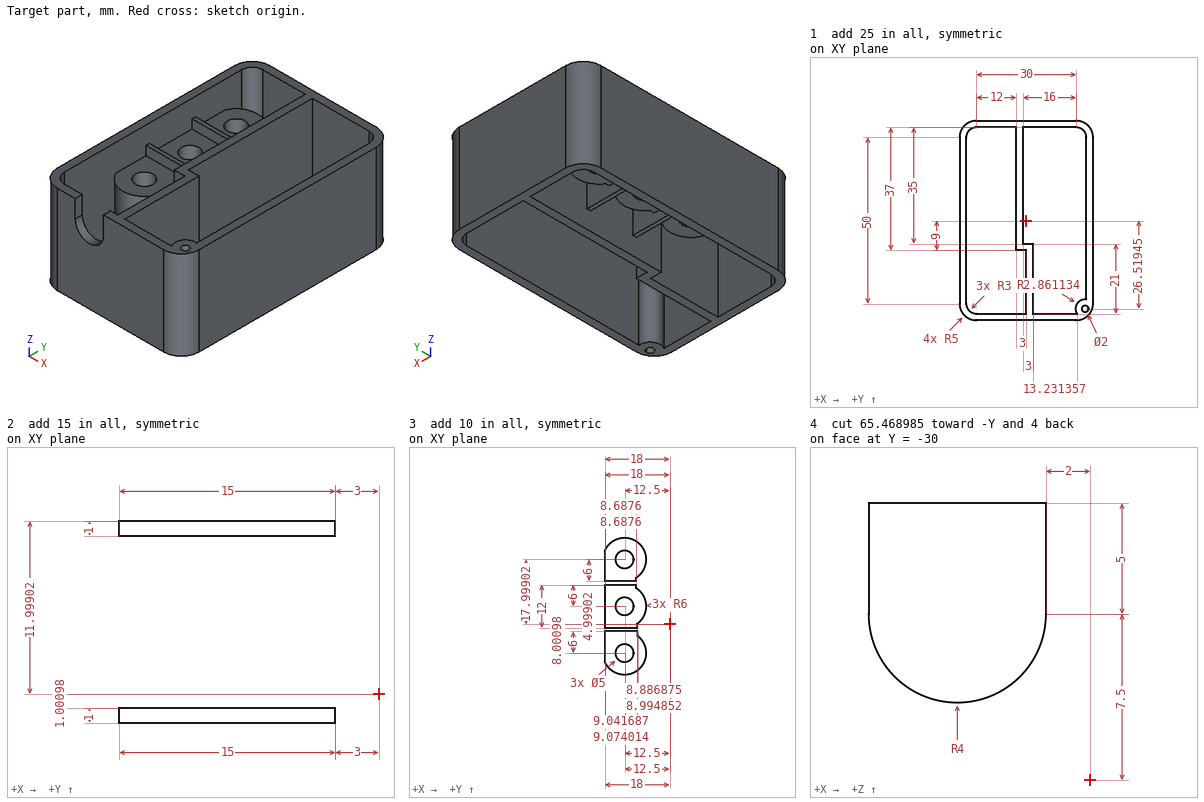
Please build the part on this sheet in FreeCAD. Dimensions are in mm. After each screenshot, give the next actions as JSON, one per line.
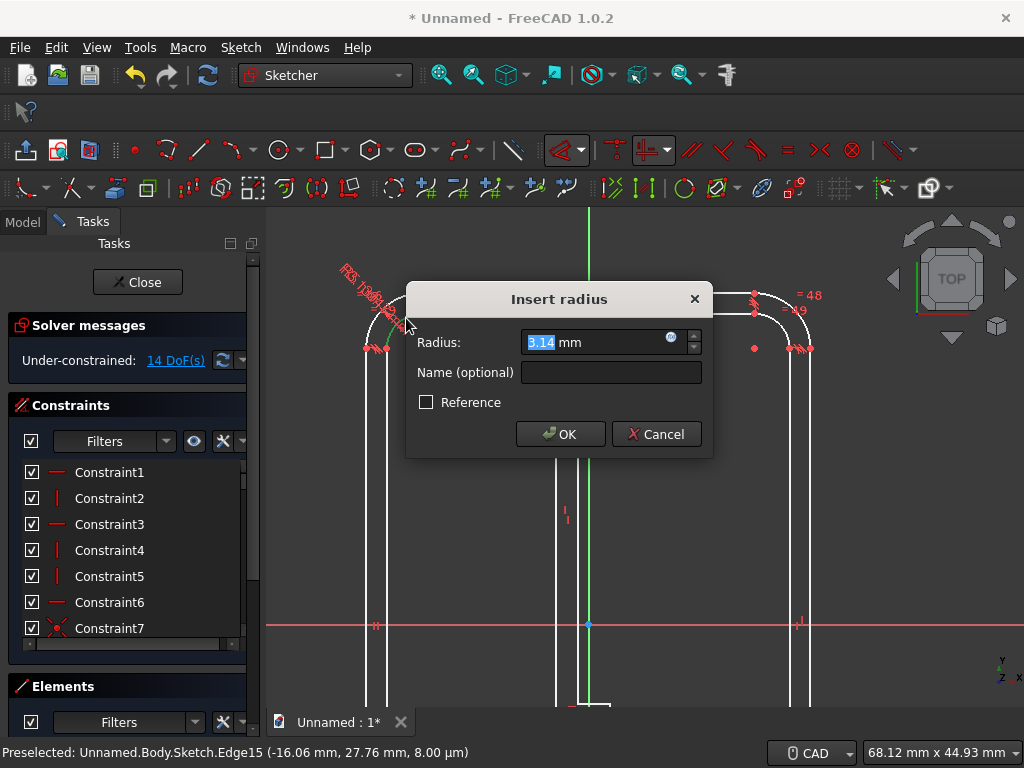
{"action": "type", "text": "3"}
{"action": "key", "text": "Return"}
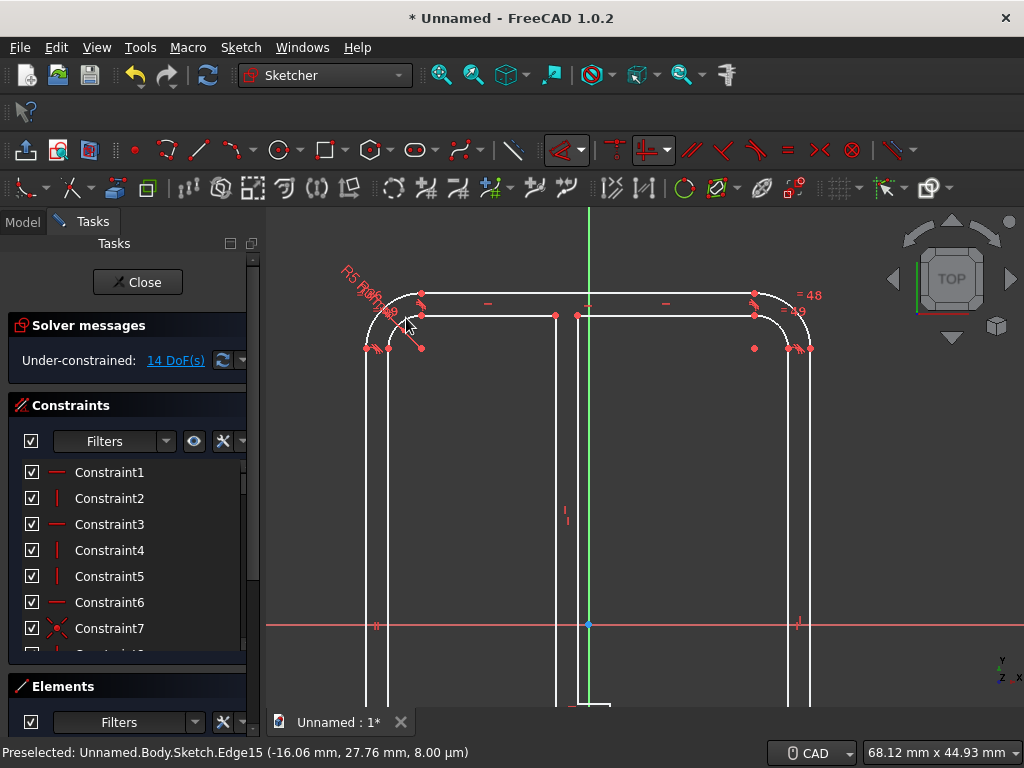
{"action": "scroll", "coordinate": [567, 320], "scroll_direction": "down", "scroll_amount": 4}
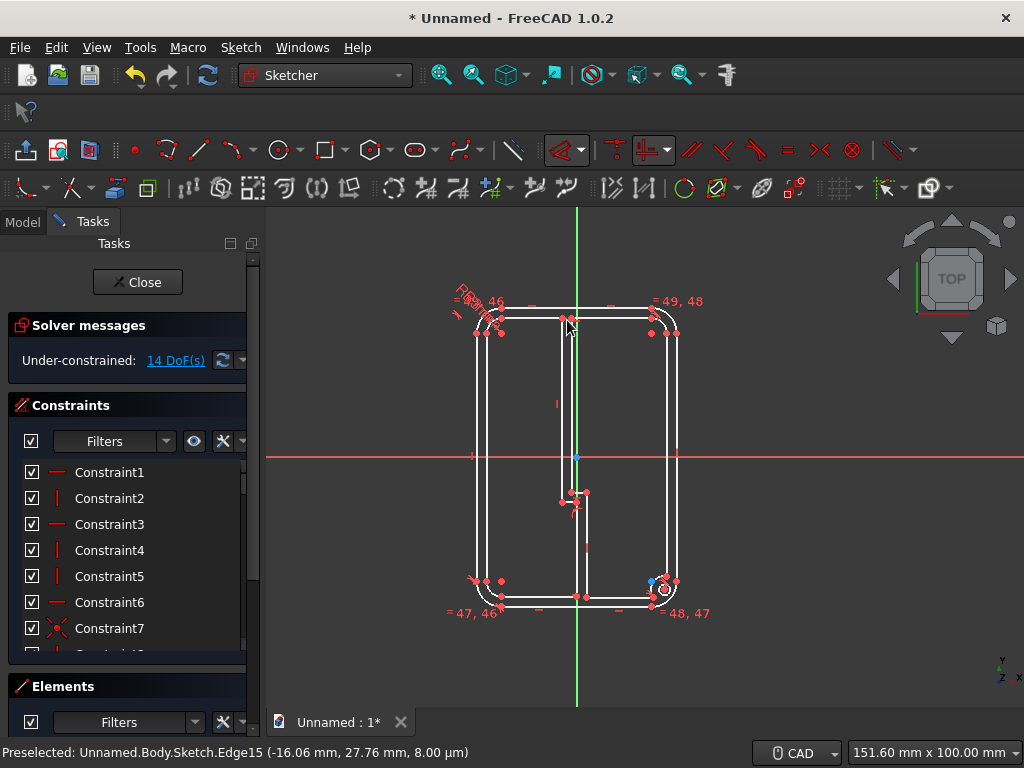
{"action": "scroll", "coordinate": [657, 578], "scroll_direction": "up", "scroll_amount": 6}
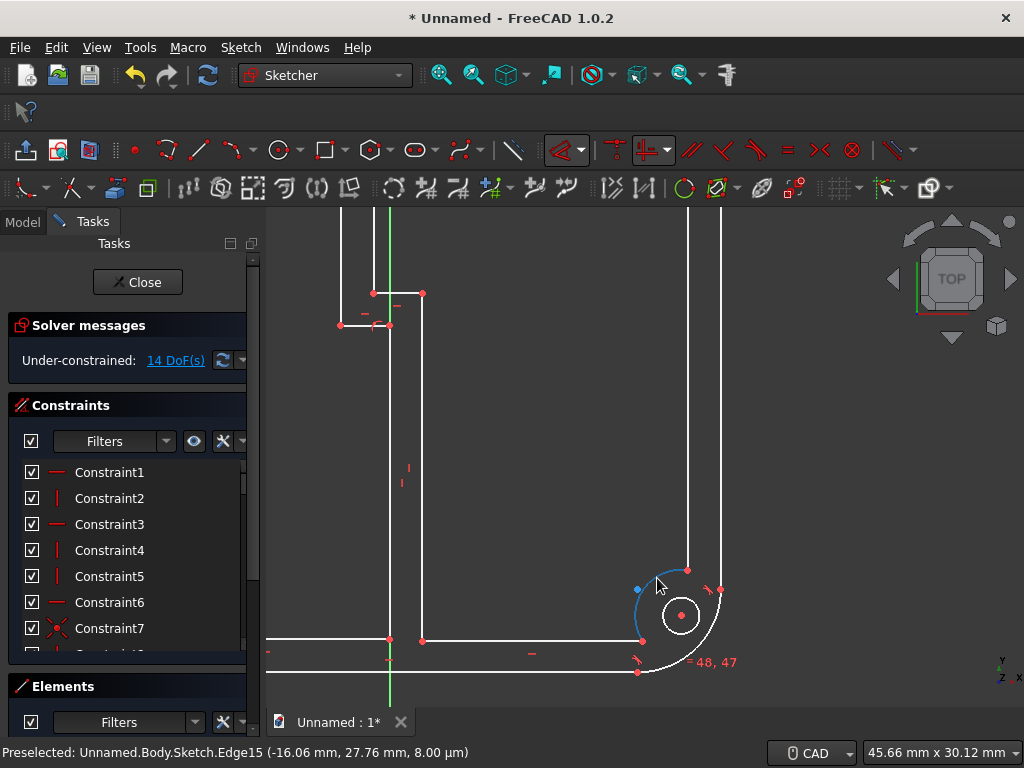
{"action": "left_click", "coordinate": [657, 577]}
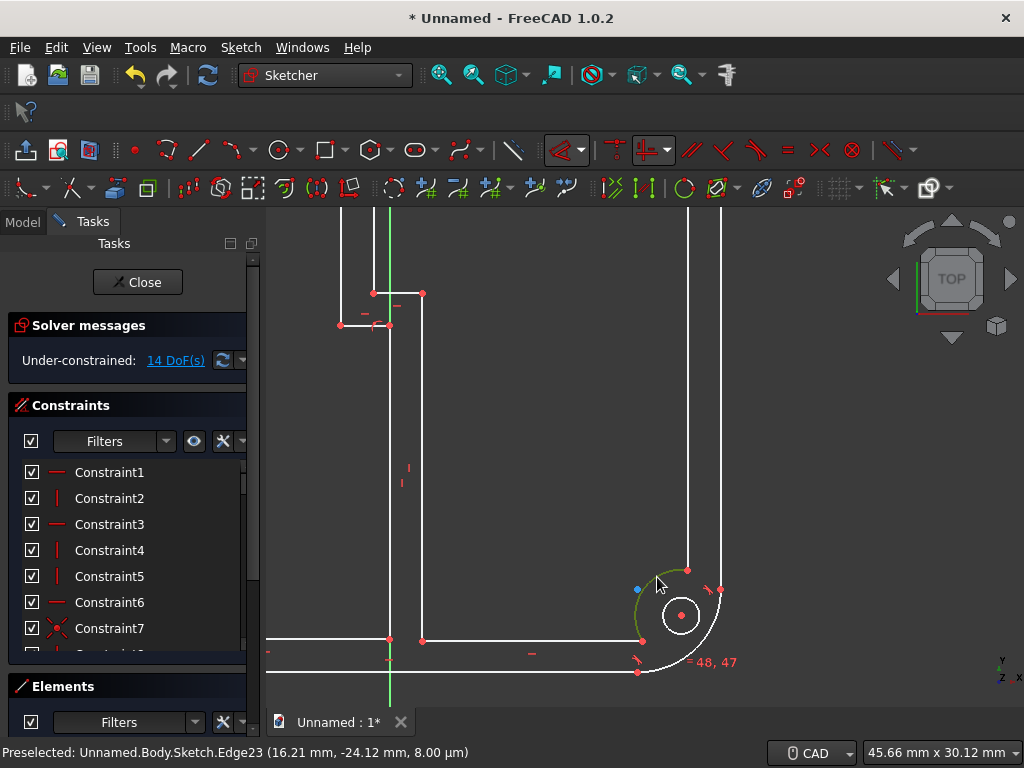
{"action": "key", "text": "k r"}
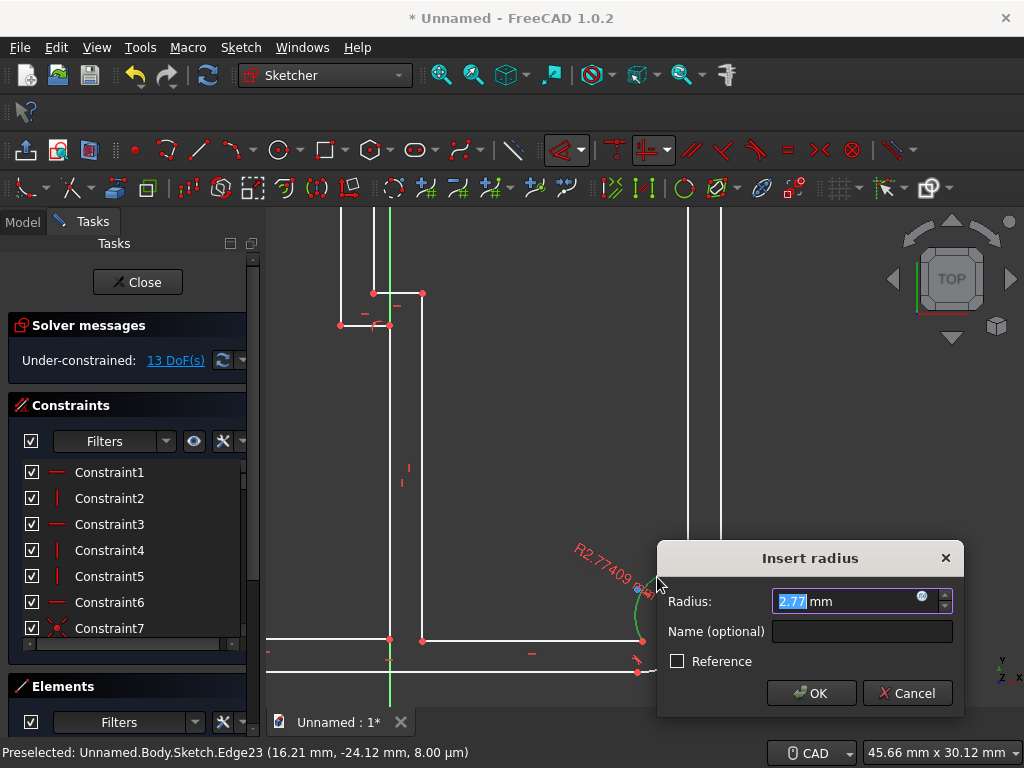
{"action": "type", "text": "2.861134"}
{"action": "key", "text": "Return"}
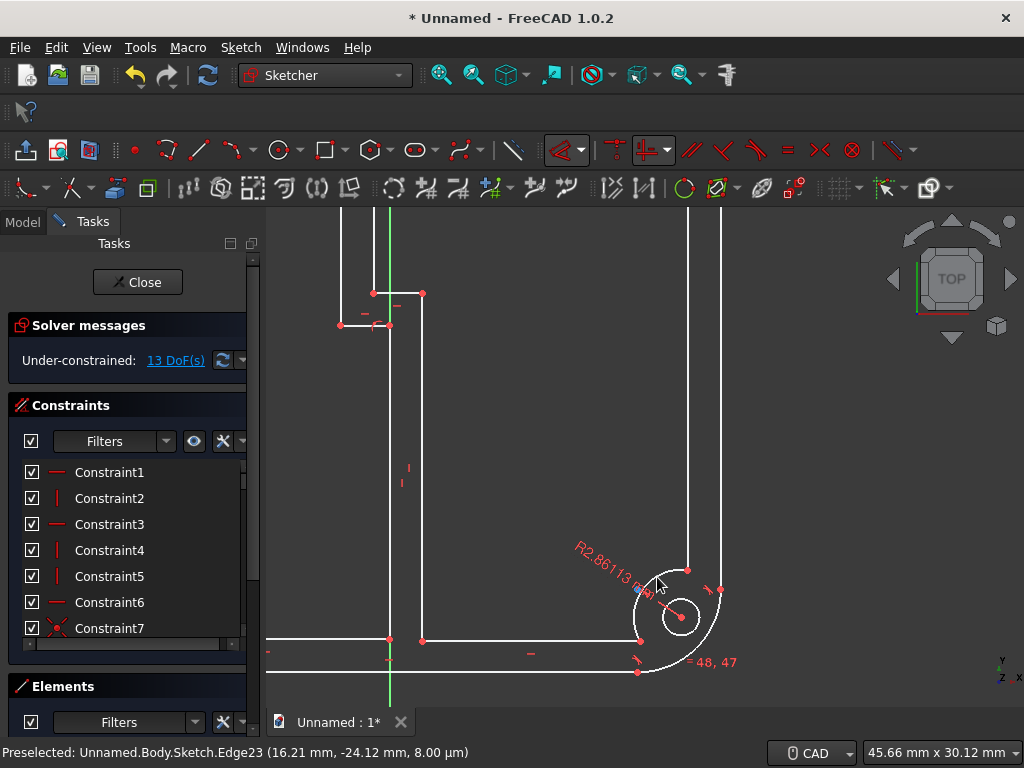
{"action": "left_click", "coordinate": [694, 604]}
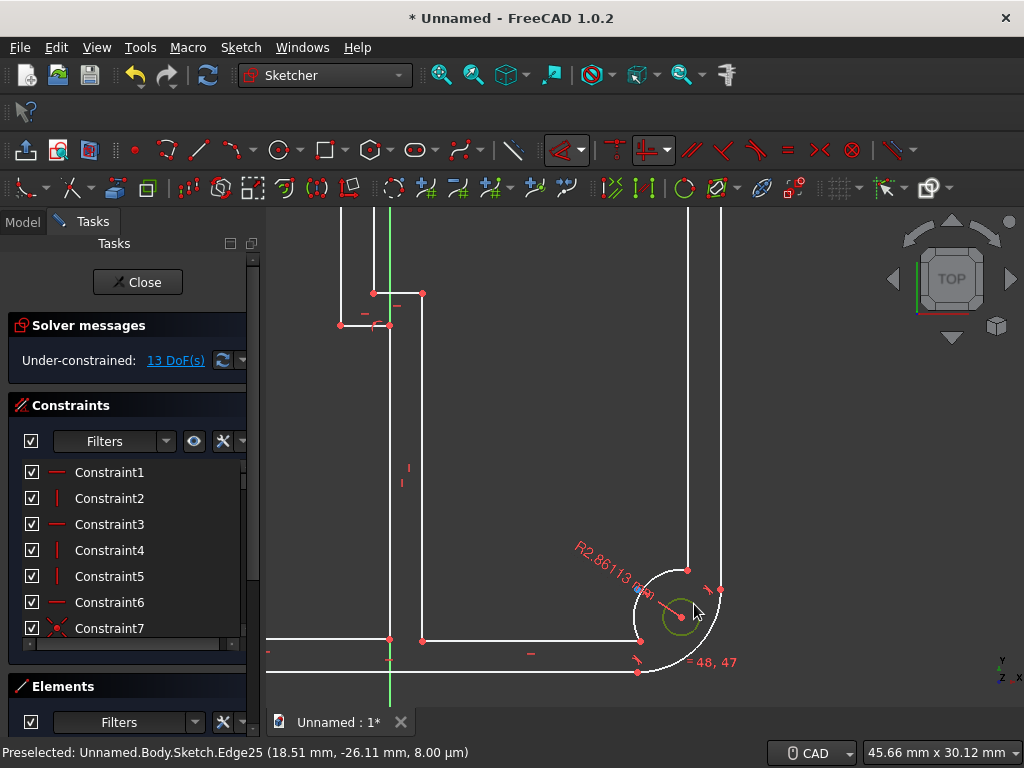
{"action": "left_click", "coordinate": [584, 150]}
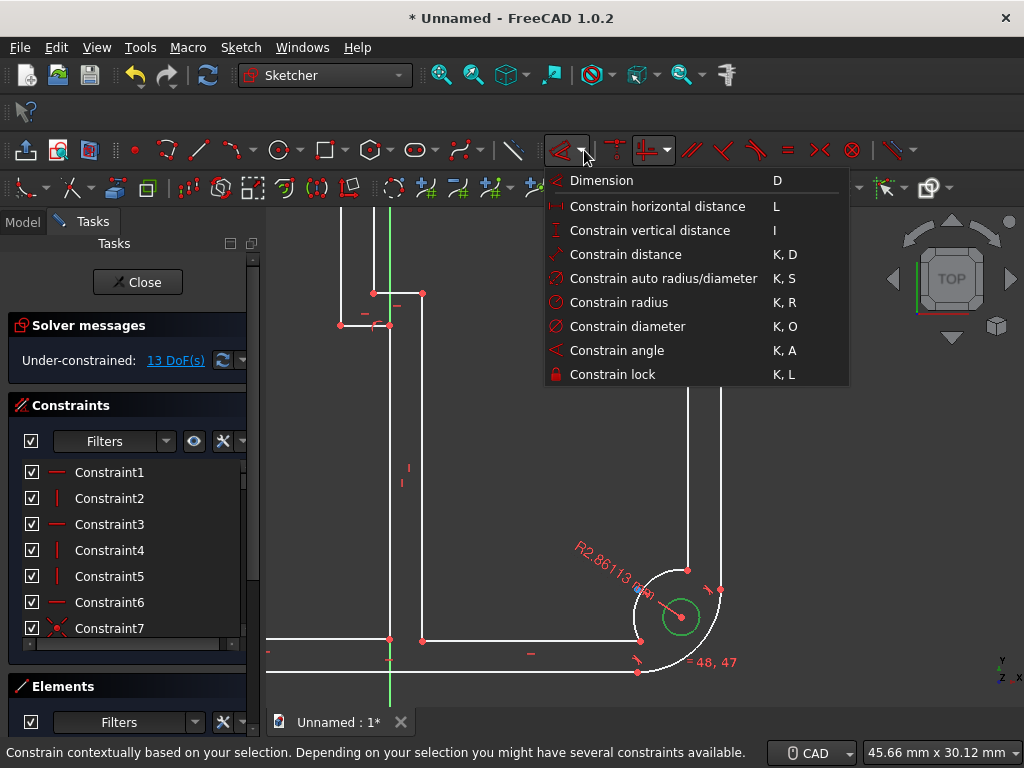
{"action": "left_click", "coordinate": [697, 326]}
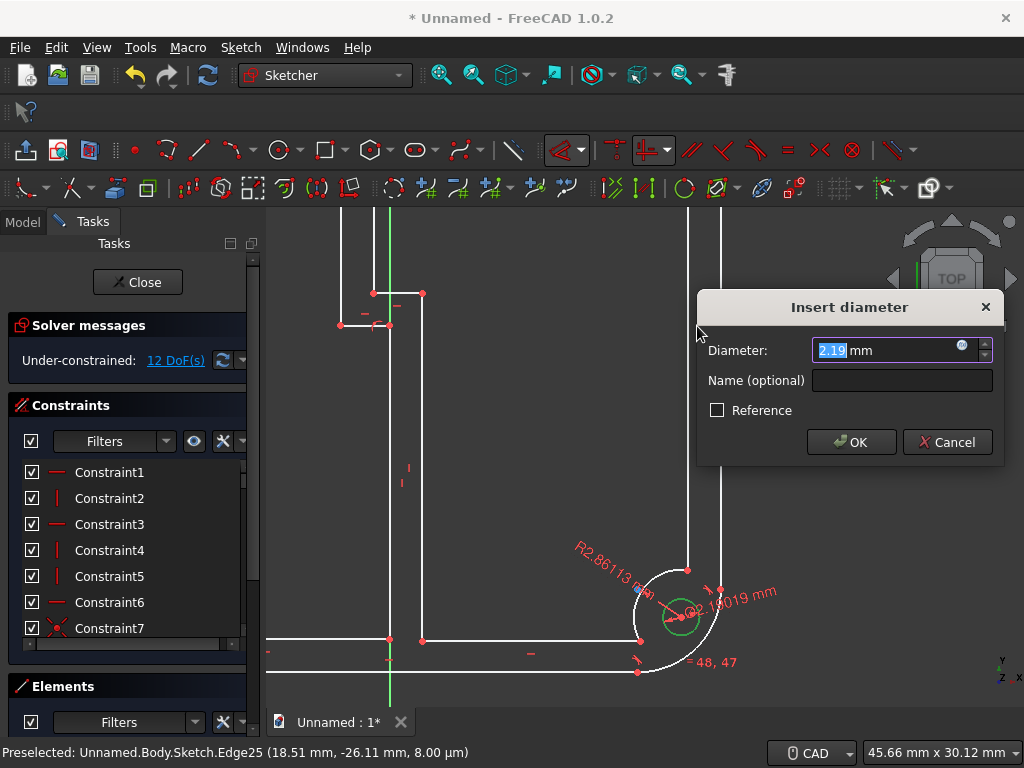
{"action": "type", "text": "2"}
{"action": "key", "text": "Return"}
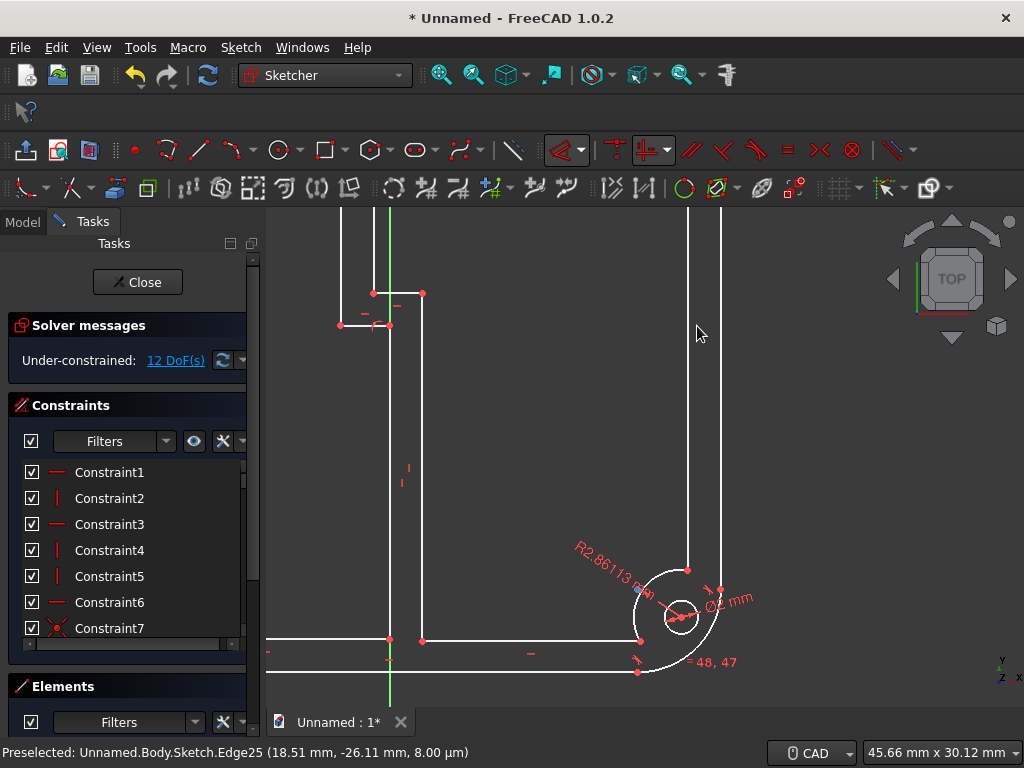
{"action": "left_click", "coordinate": [355, 326]}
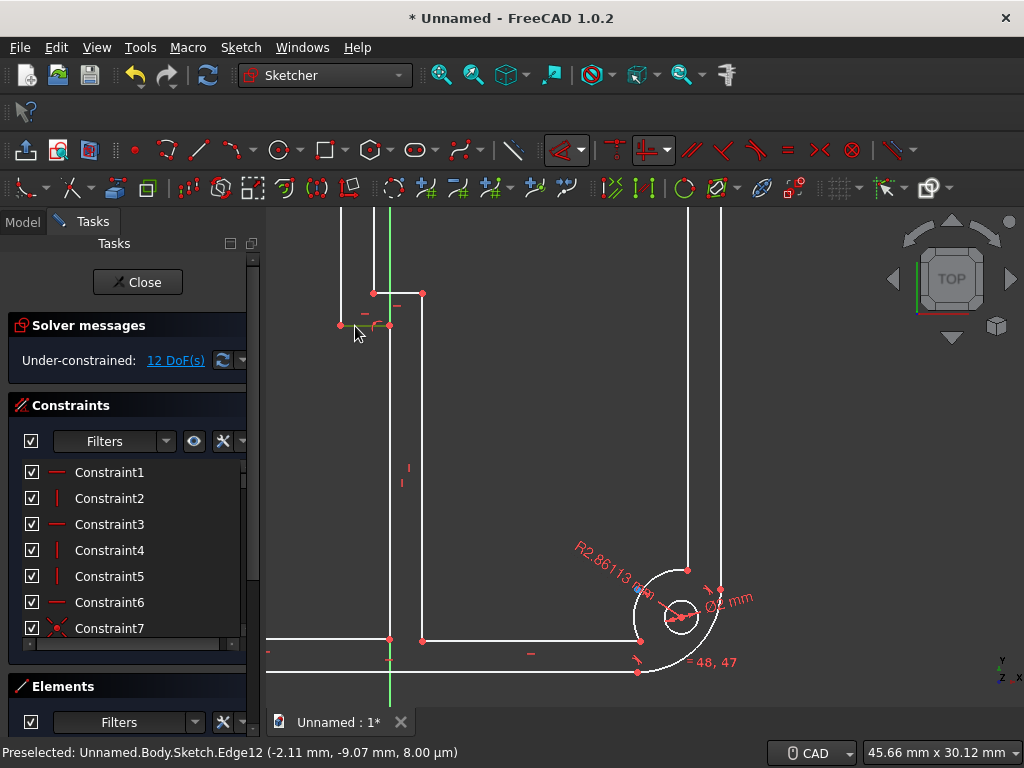
{"action": "key", "text": "l"}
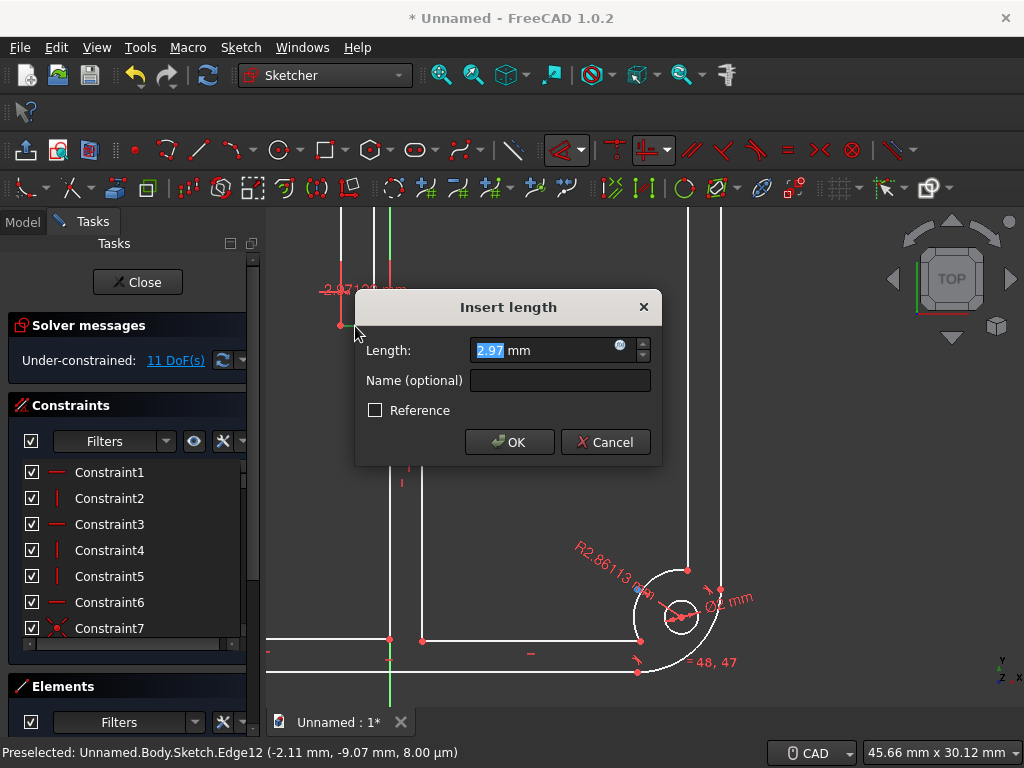
{"action": "type", "text": "3"}
{"action": "key", "text": "Return"}